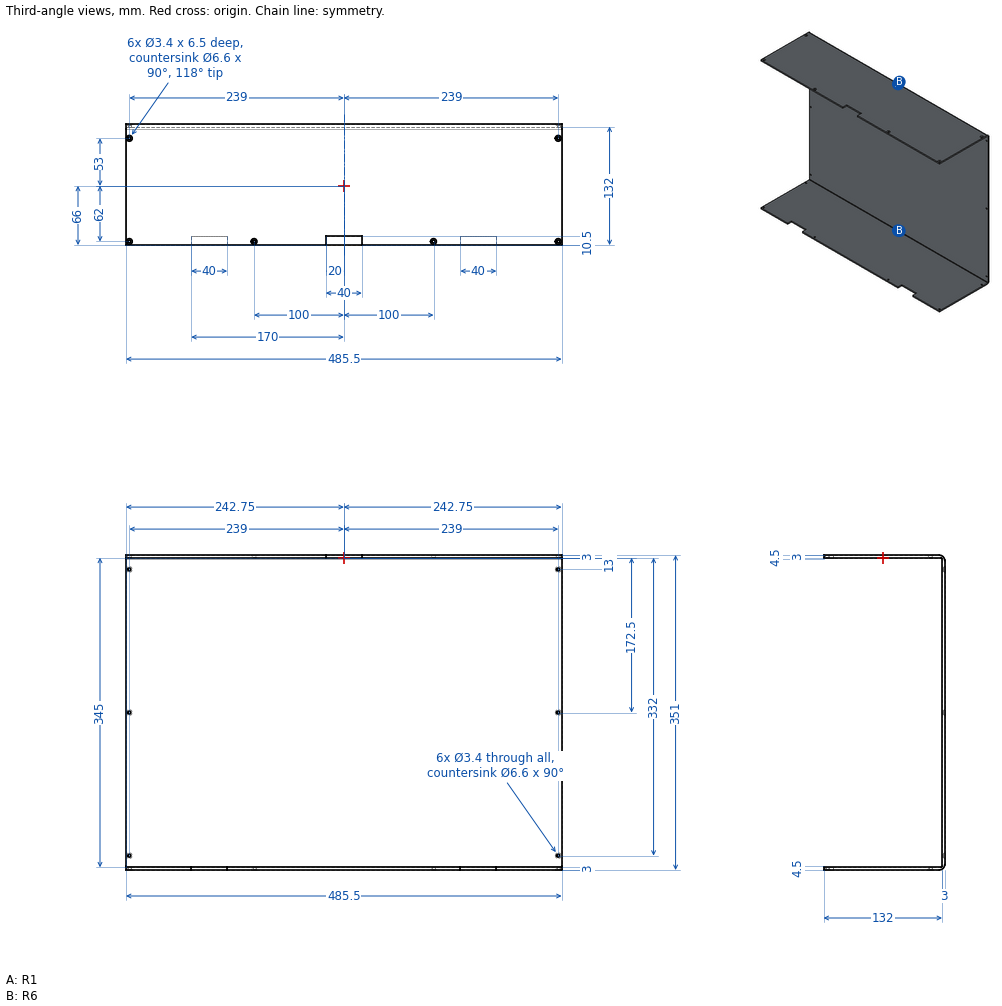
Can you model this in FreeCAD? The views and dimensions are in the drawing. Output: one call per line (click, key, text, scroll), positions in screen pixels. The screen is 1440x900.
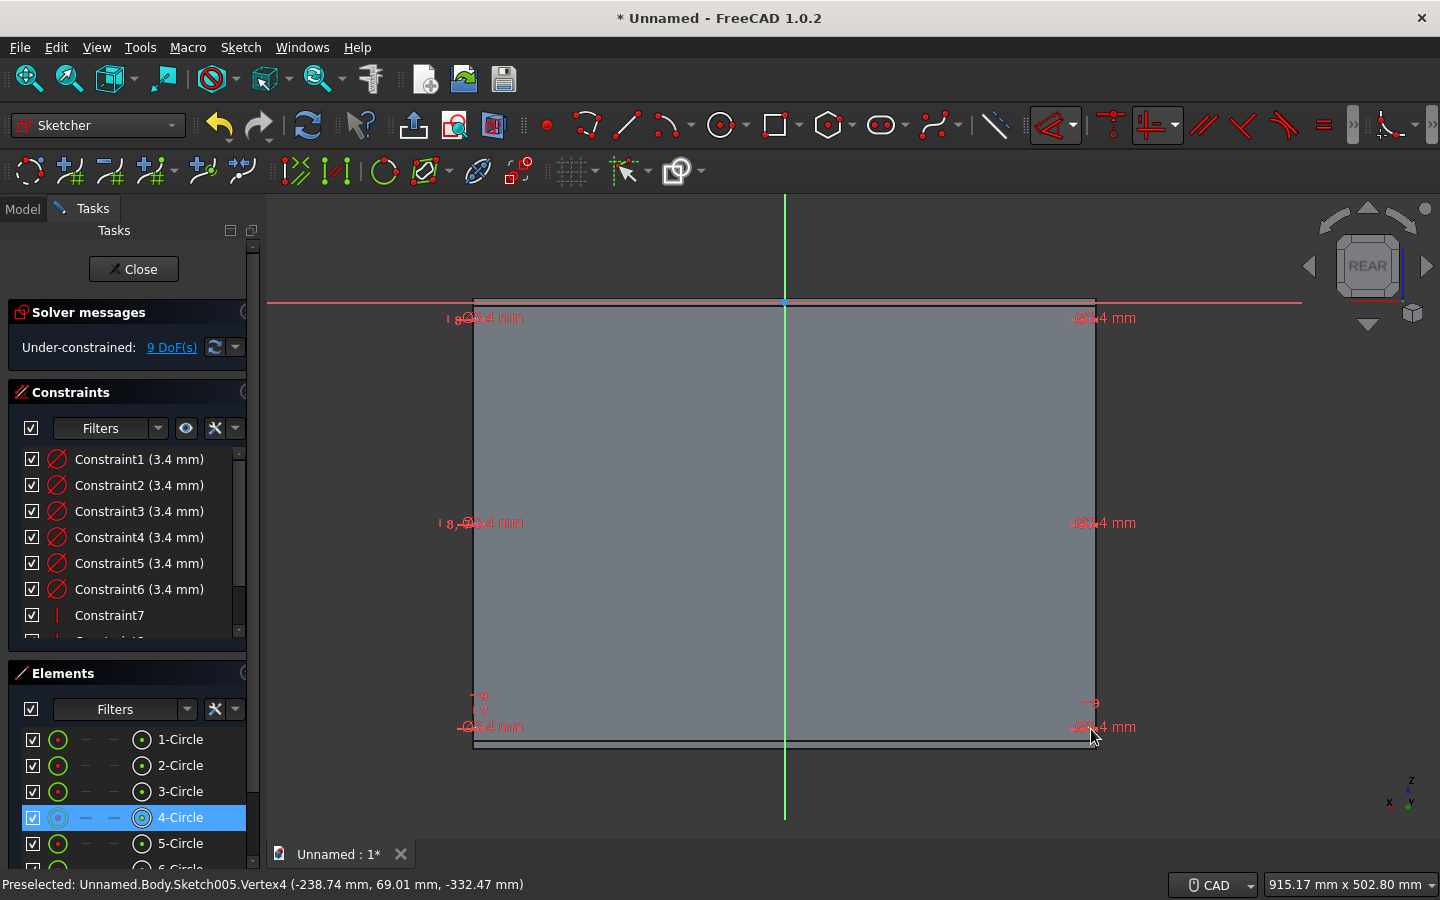
click(1091, 525)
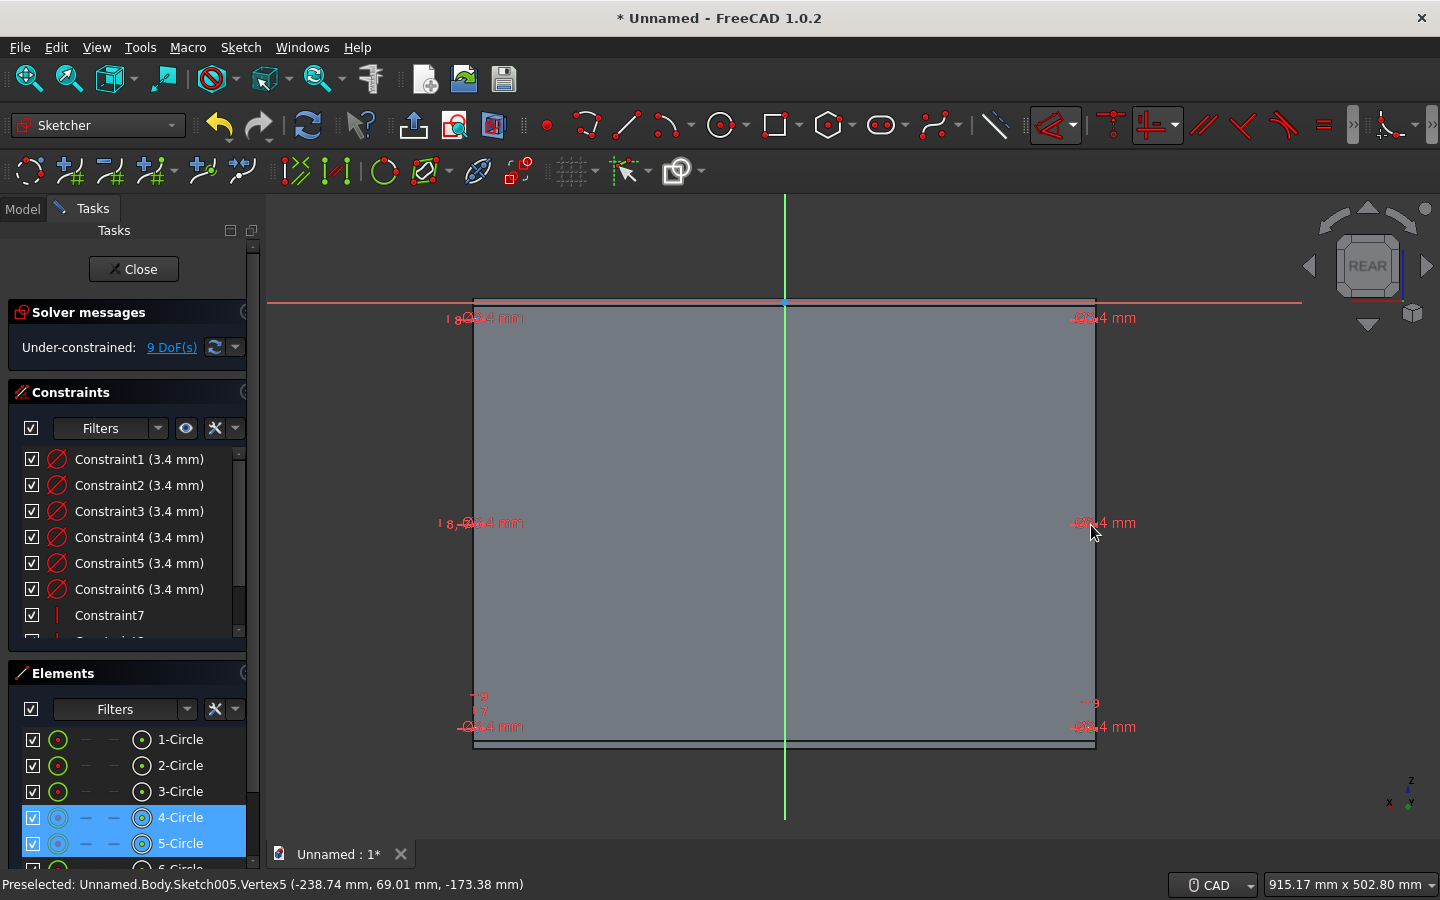
key(v)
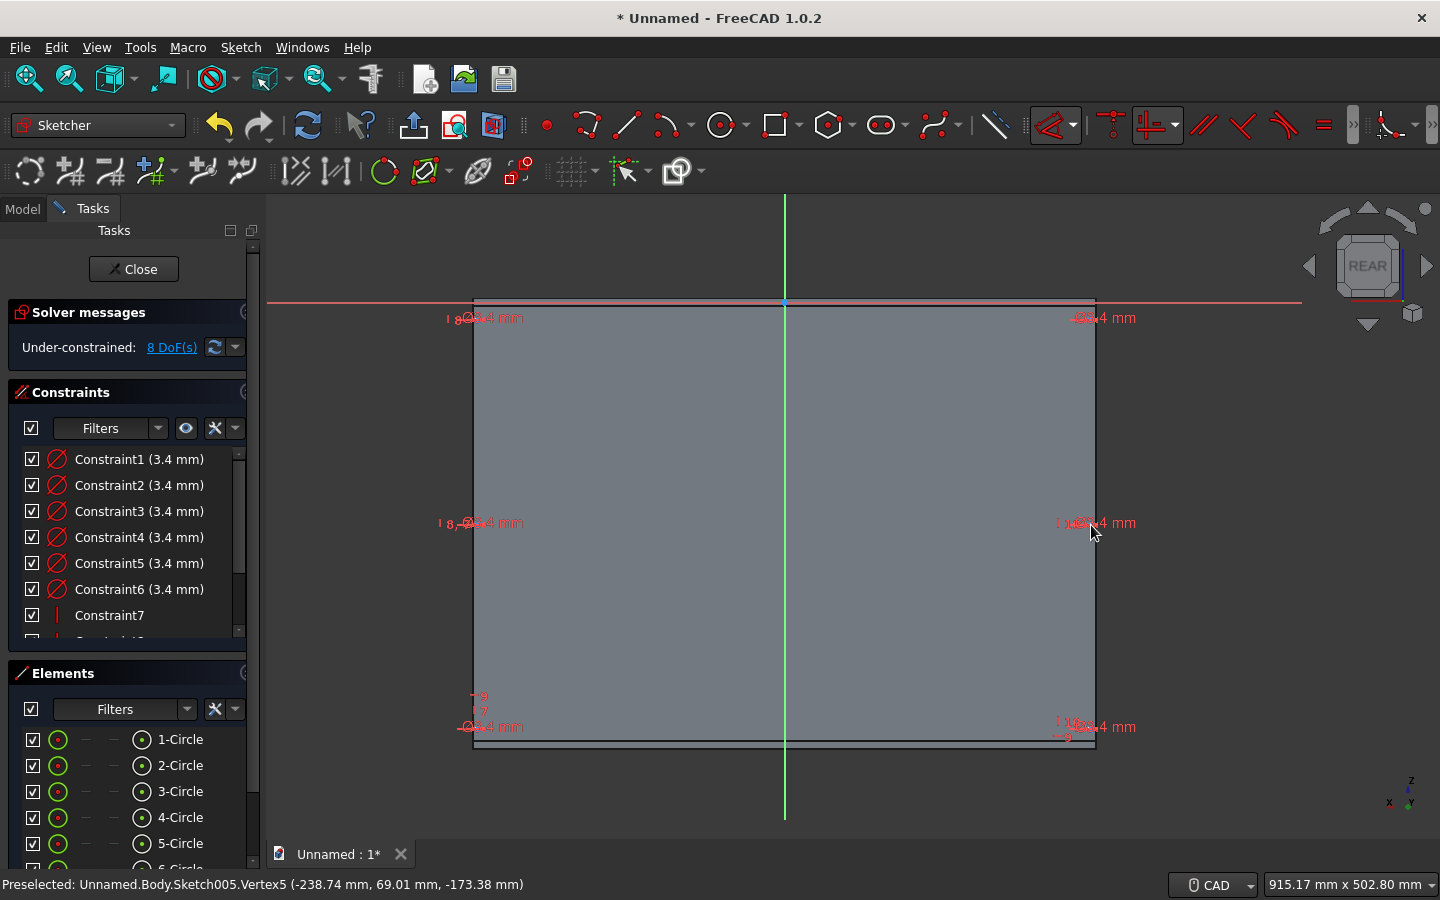
click(478, 525)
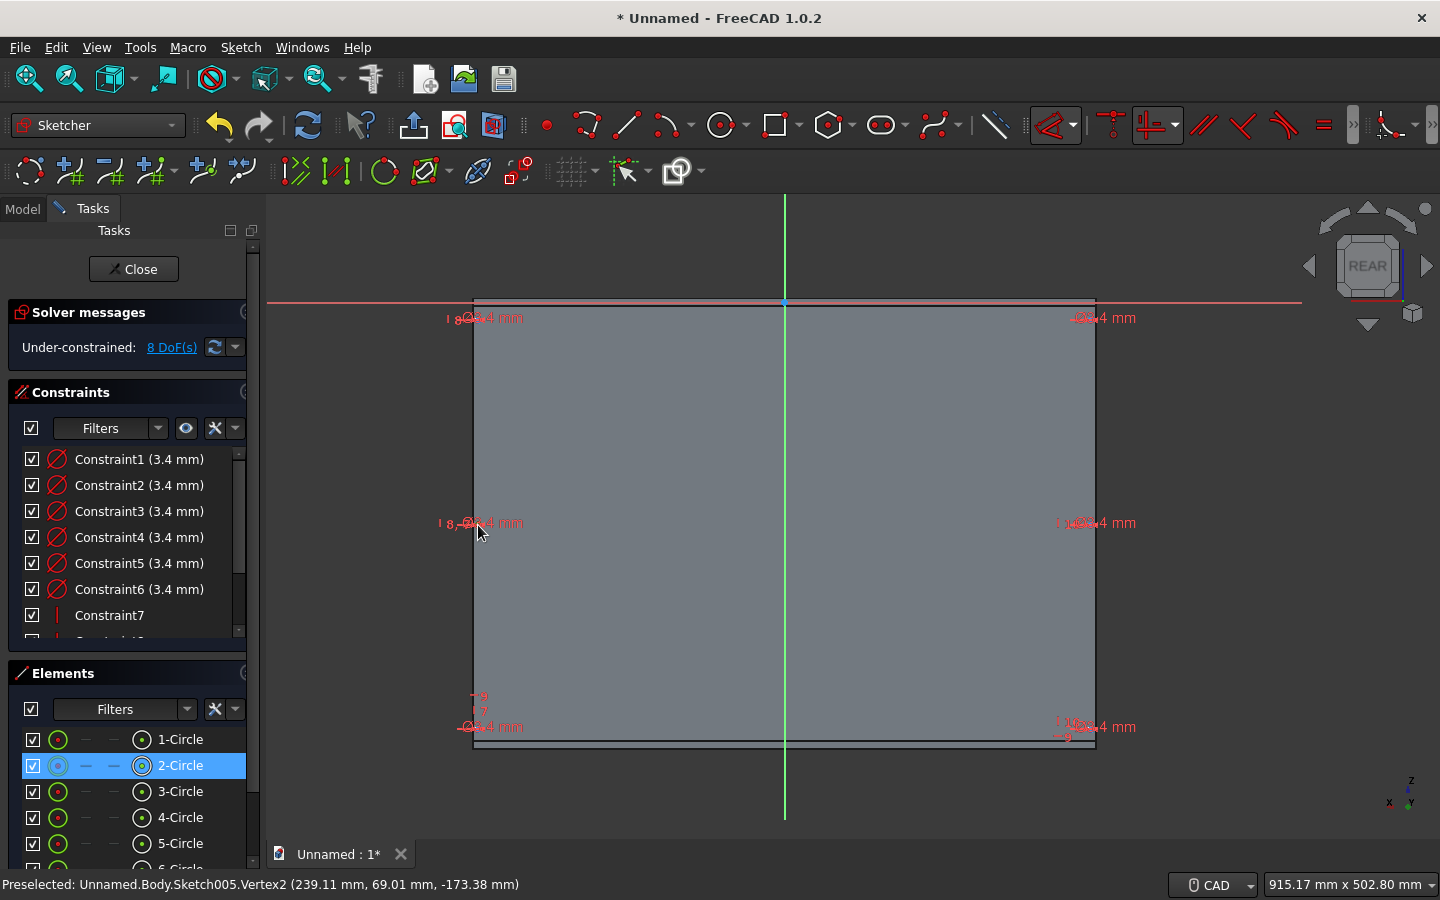
click(1091, 525)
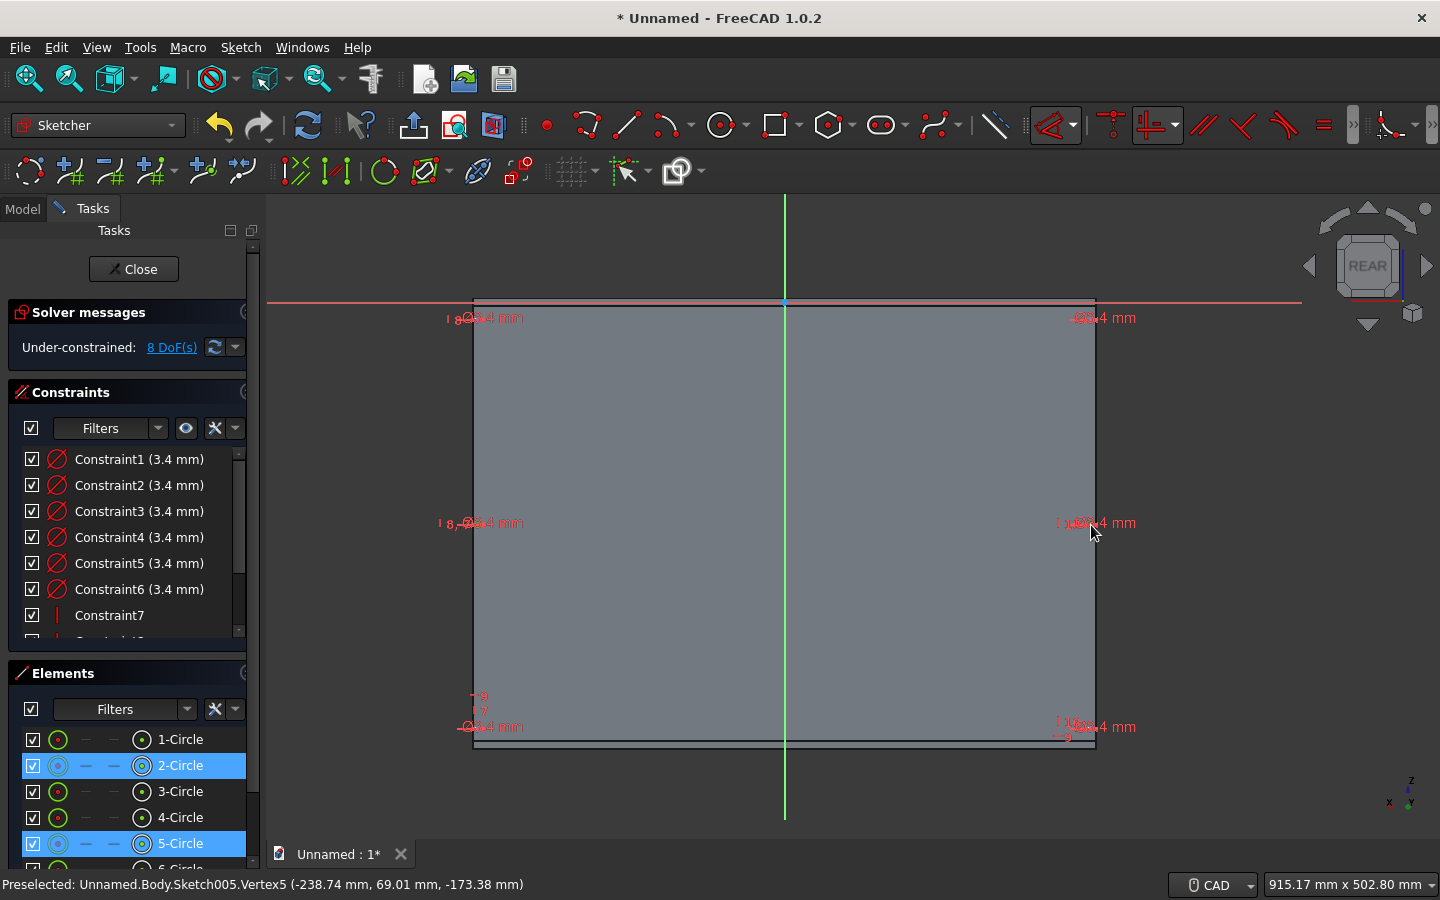
click(1178, 126)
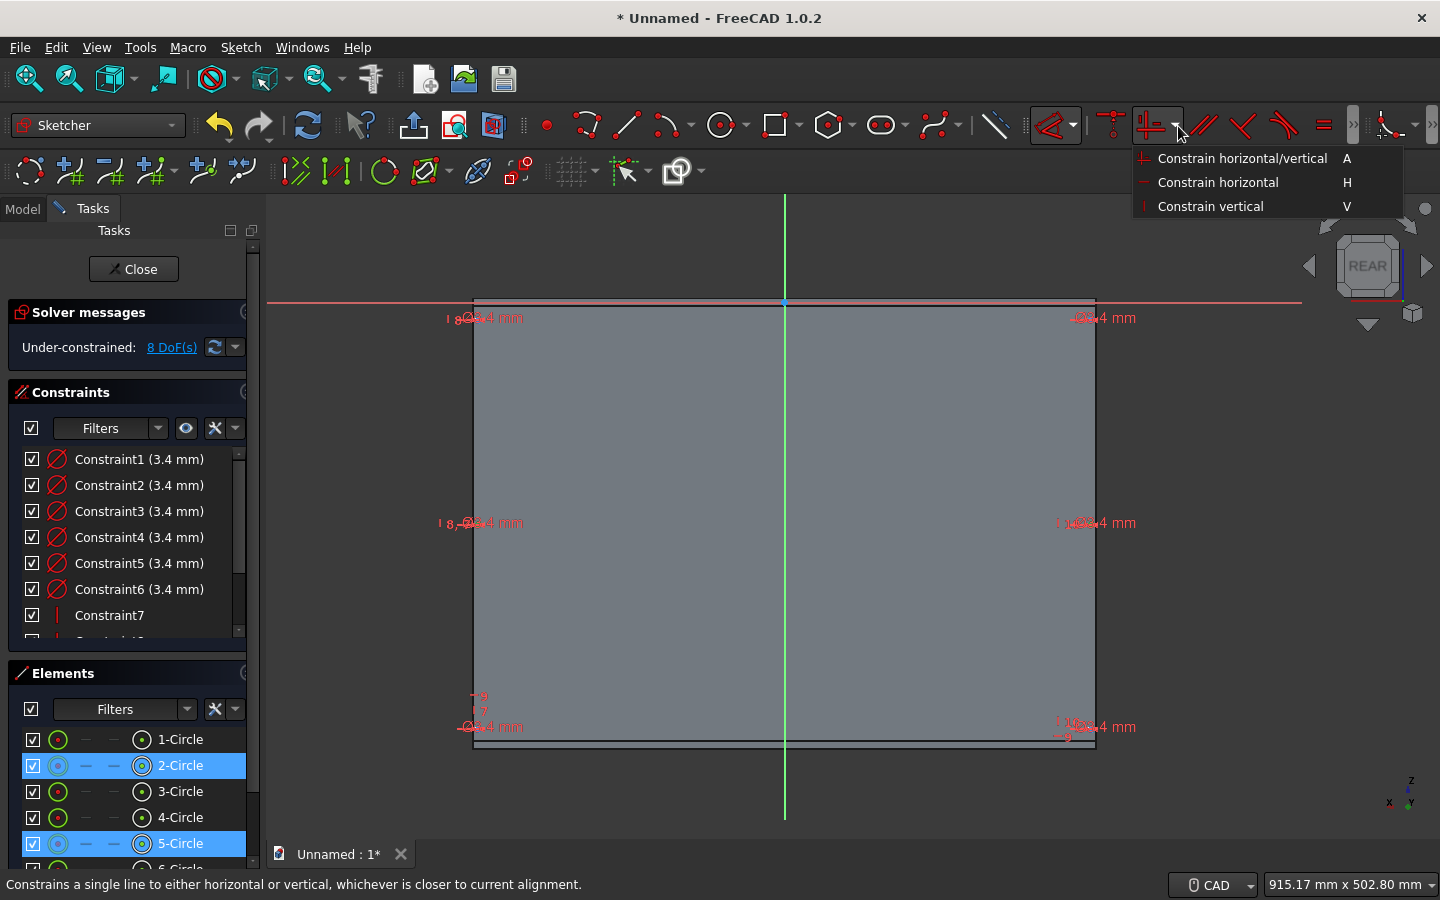
click(1268, 182)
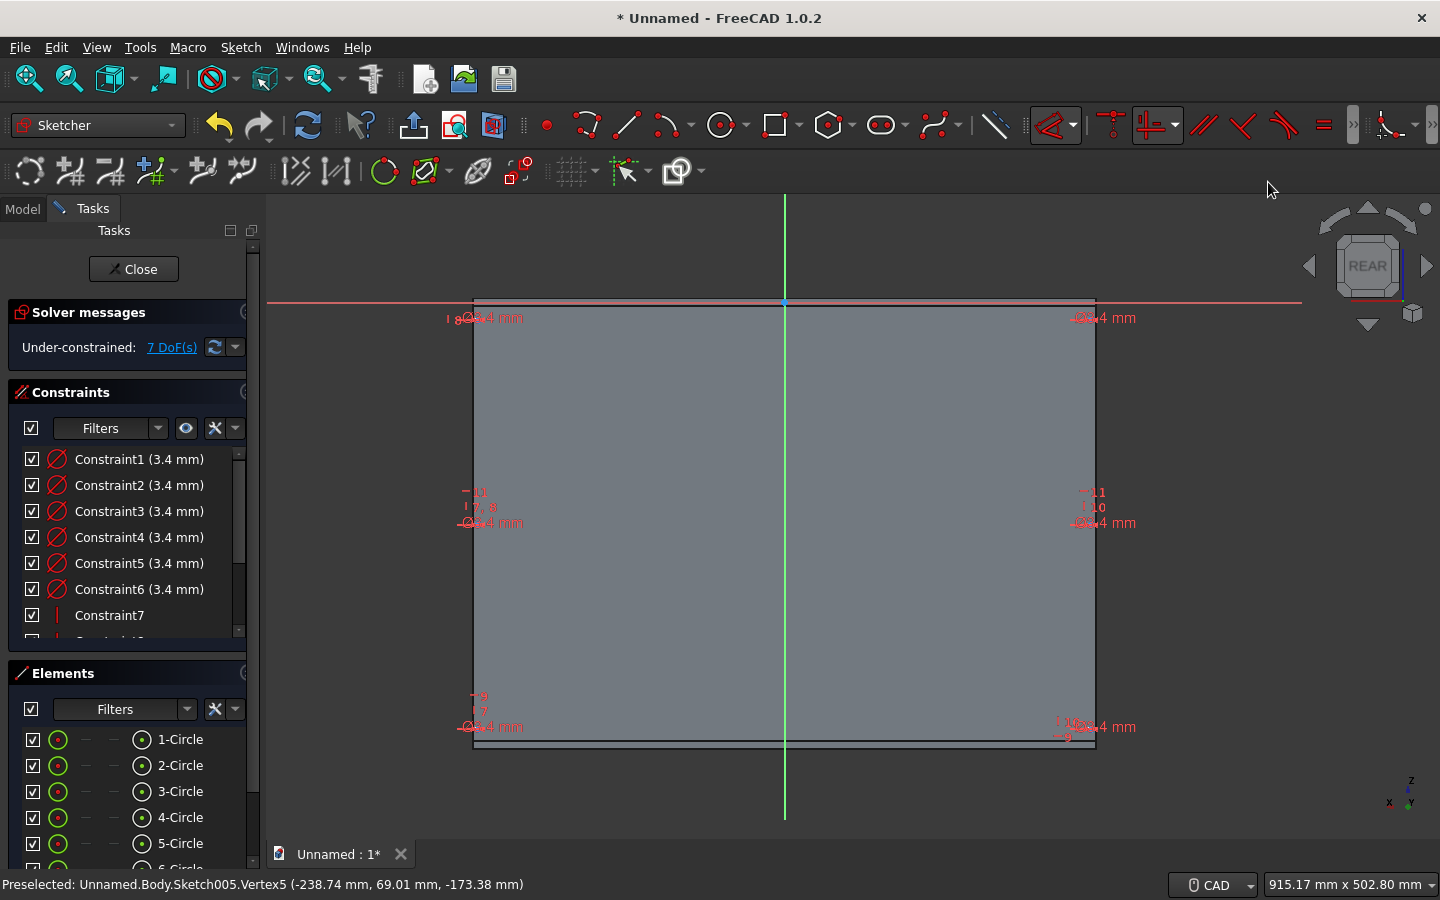
click(1091, 525)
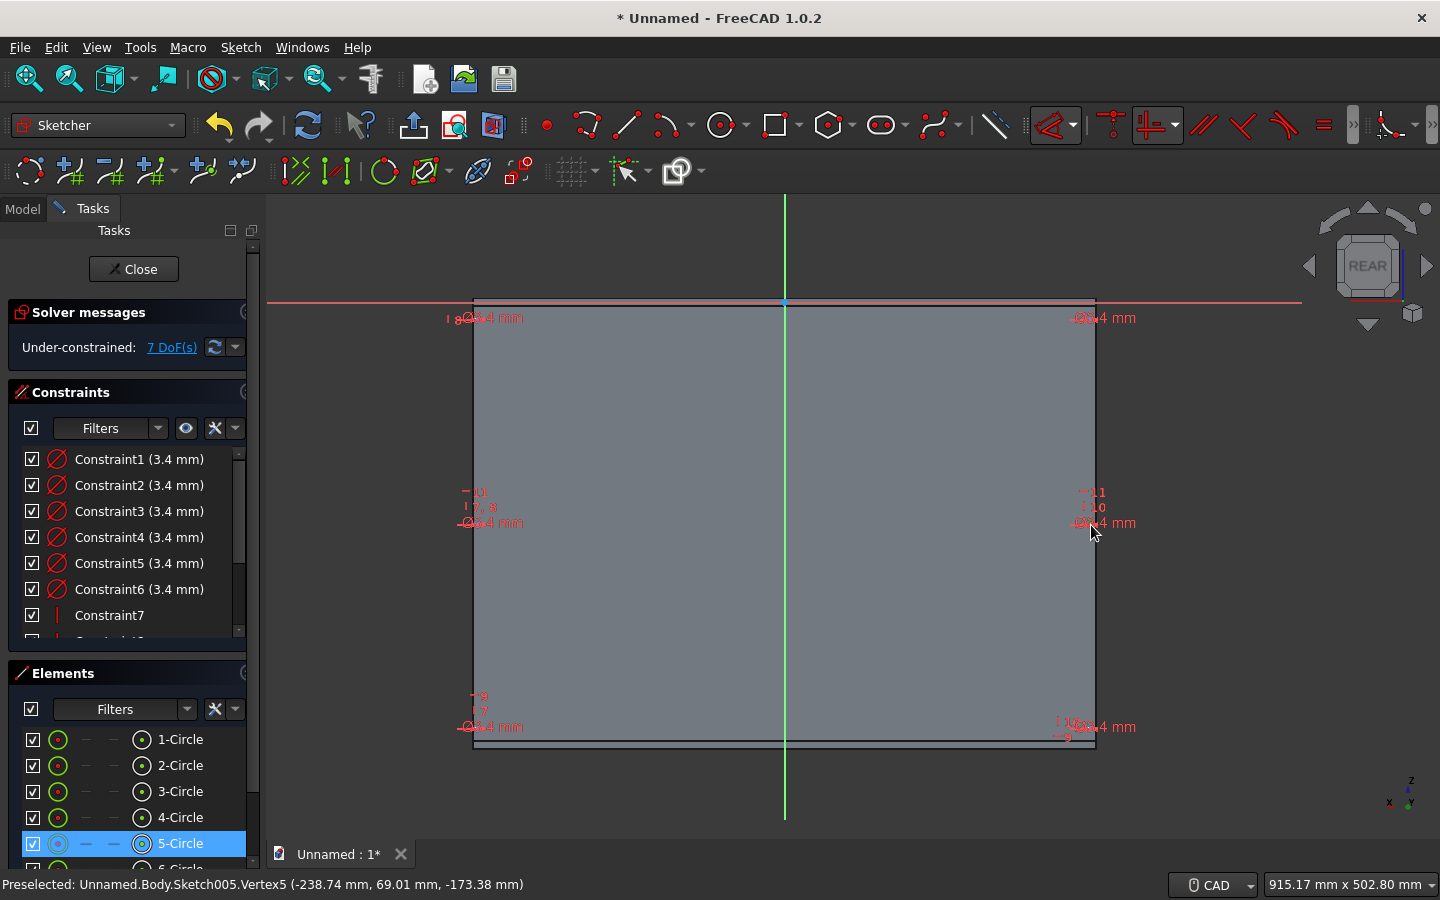
click(1091, 320)